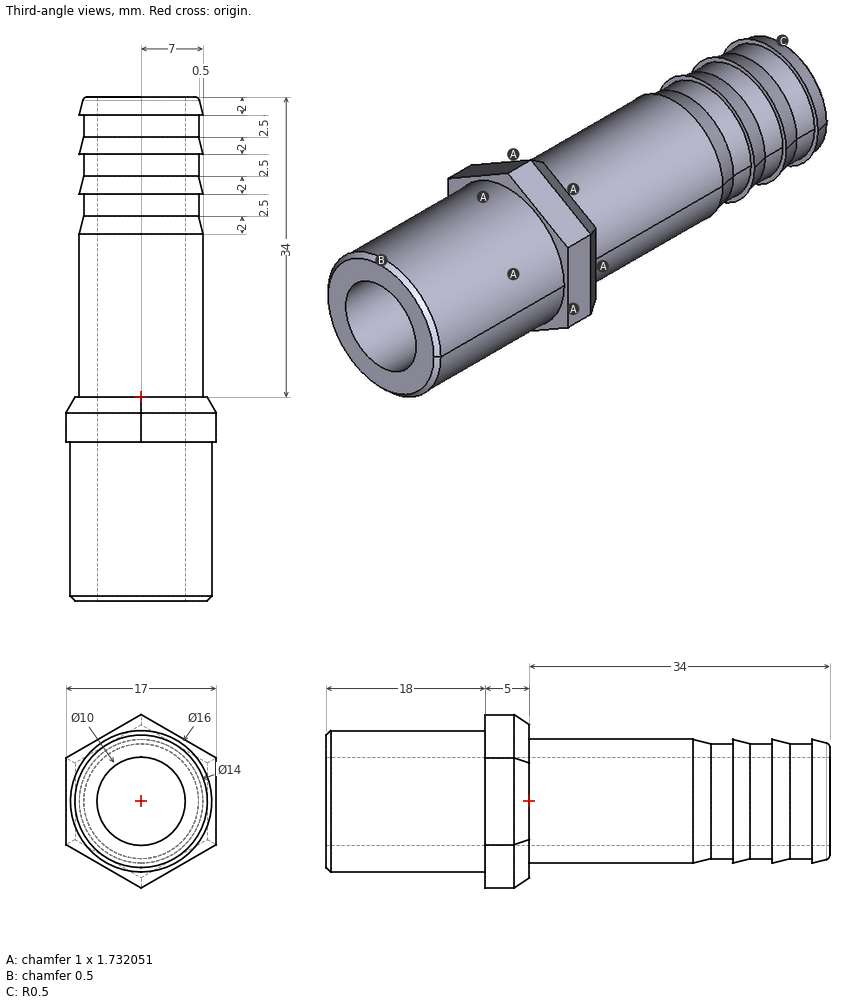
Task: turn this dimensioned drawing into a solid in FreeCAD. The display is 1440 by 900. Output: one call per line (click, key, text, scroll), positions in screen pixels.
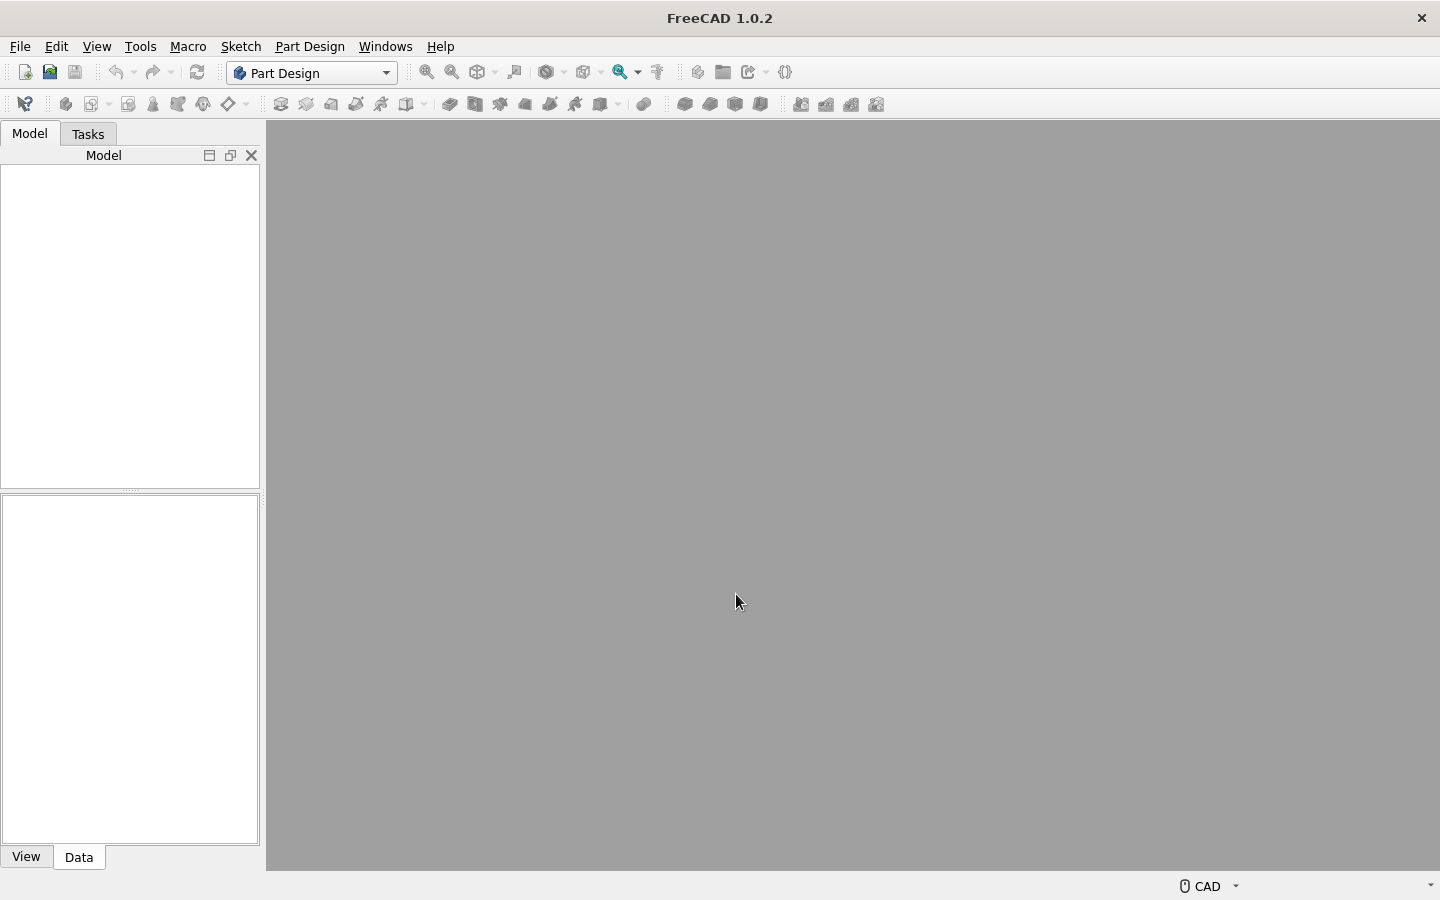
click(25, 72)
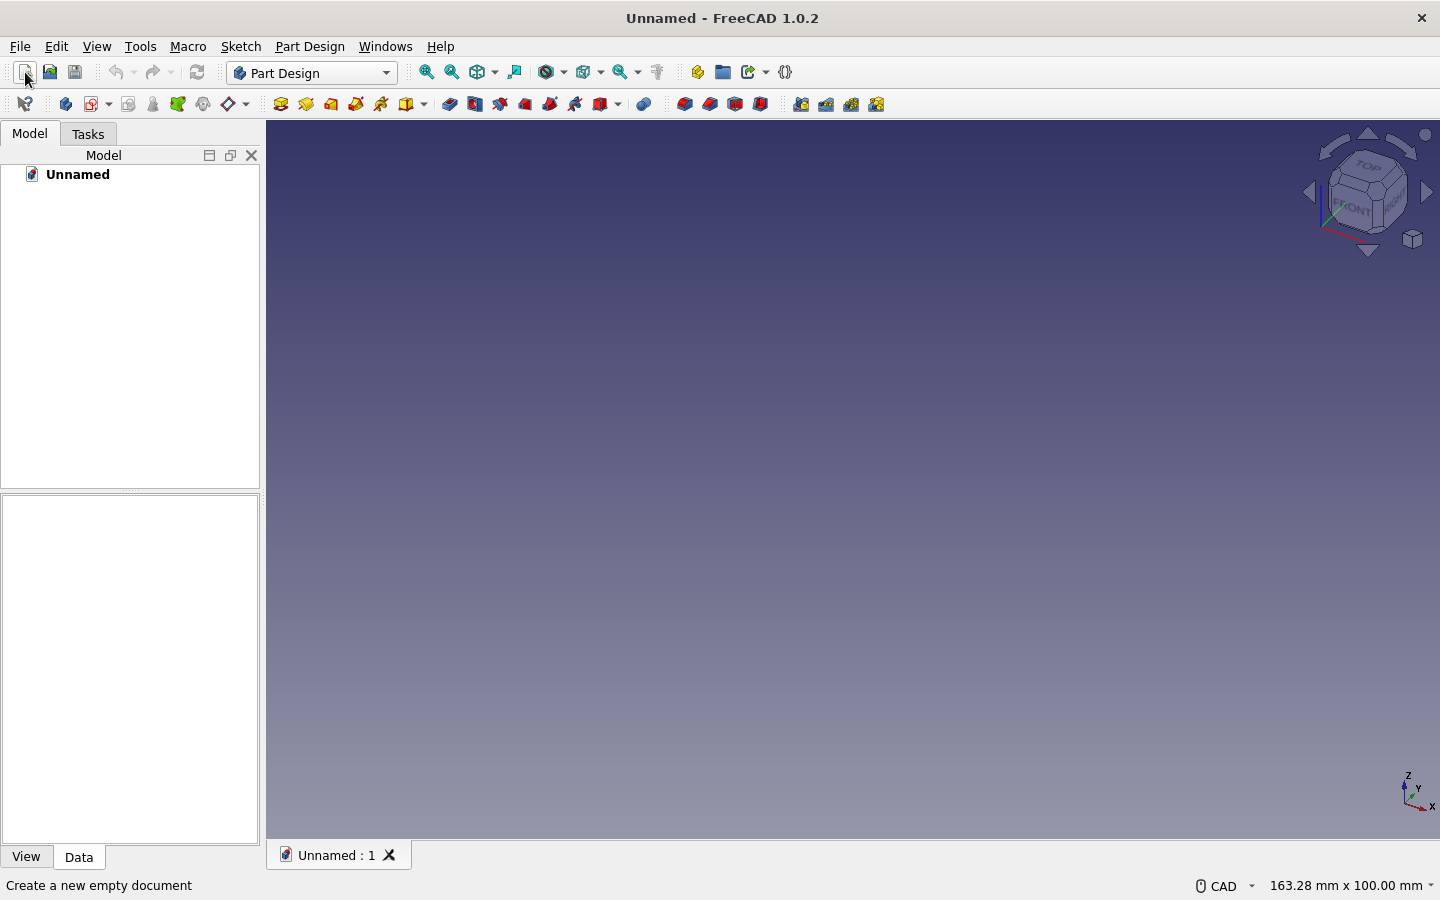
click(90, 104)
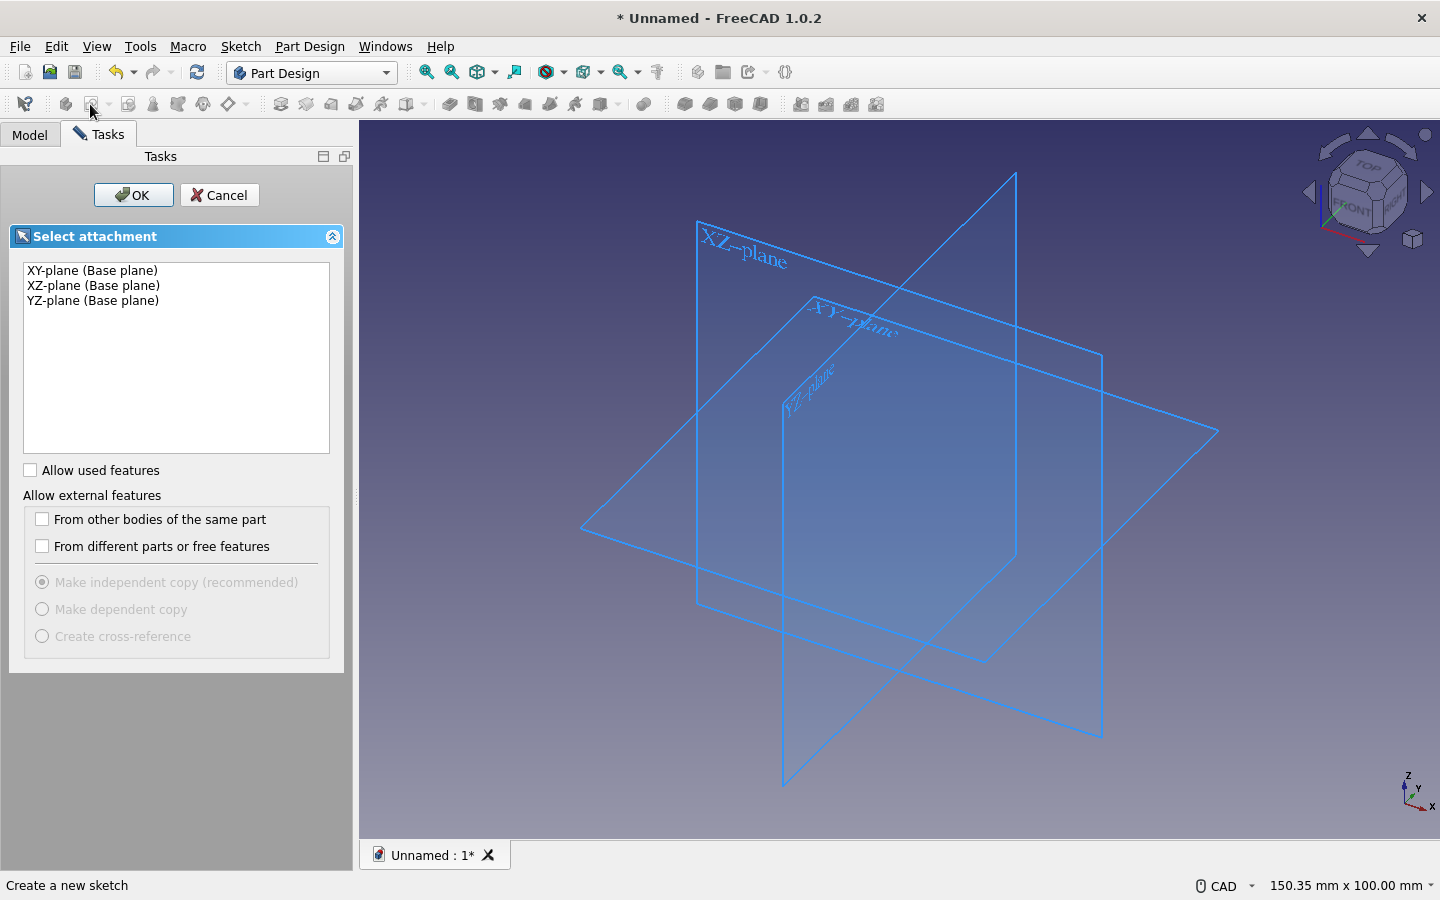
click(84, 286)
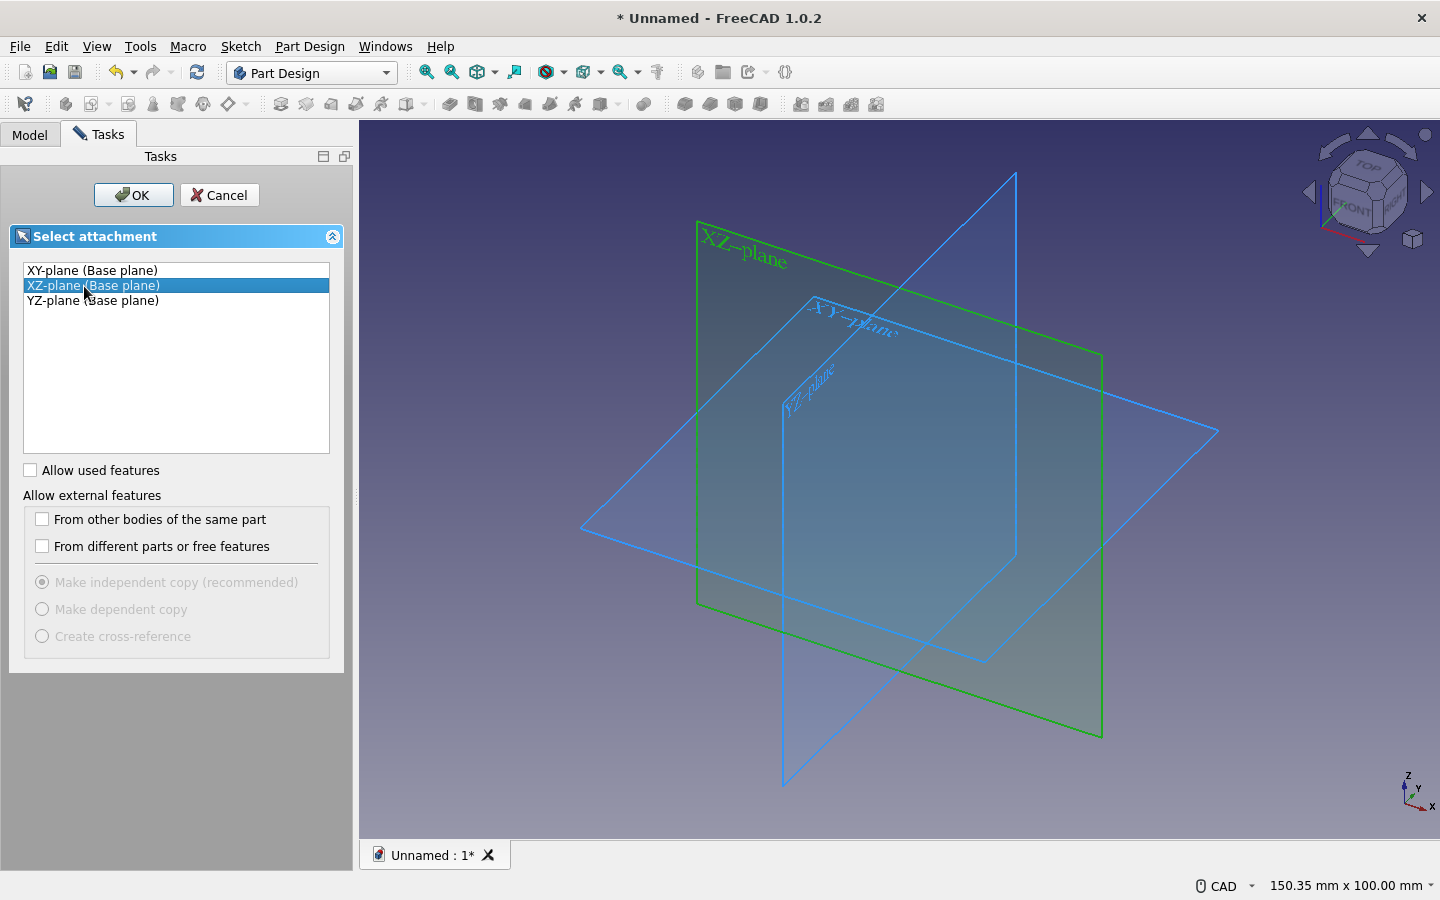
click(134, 195)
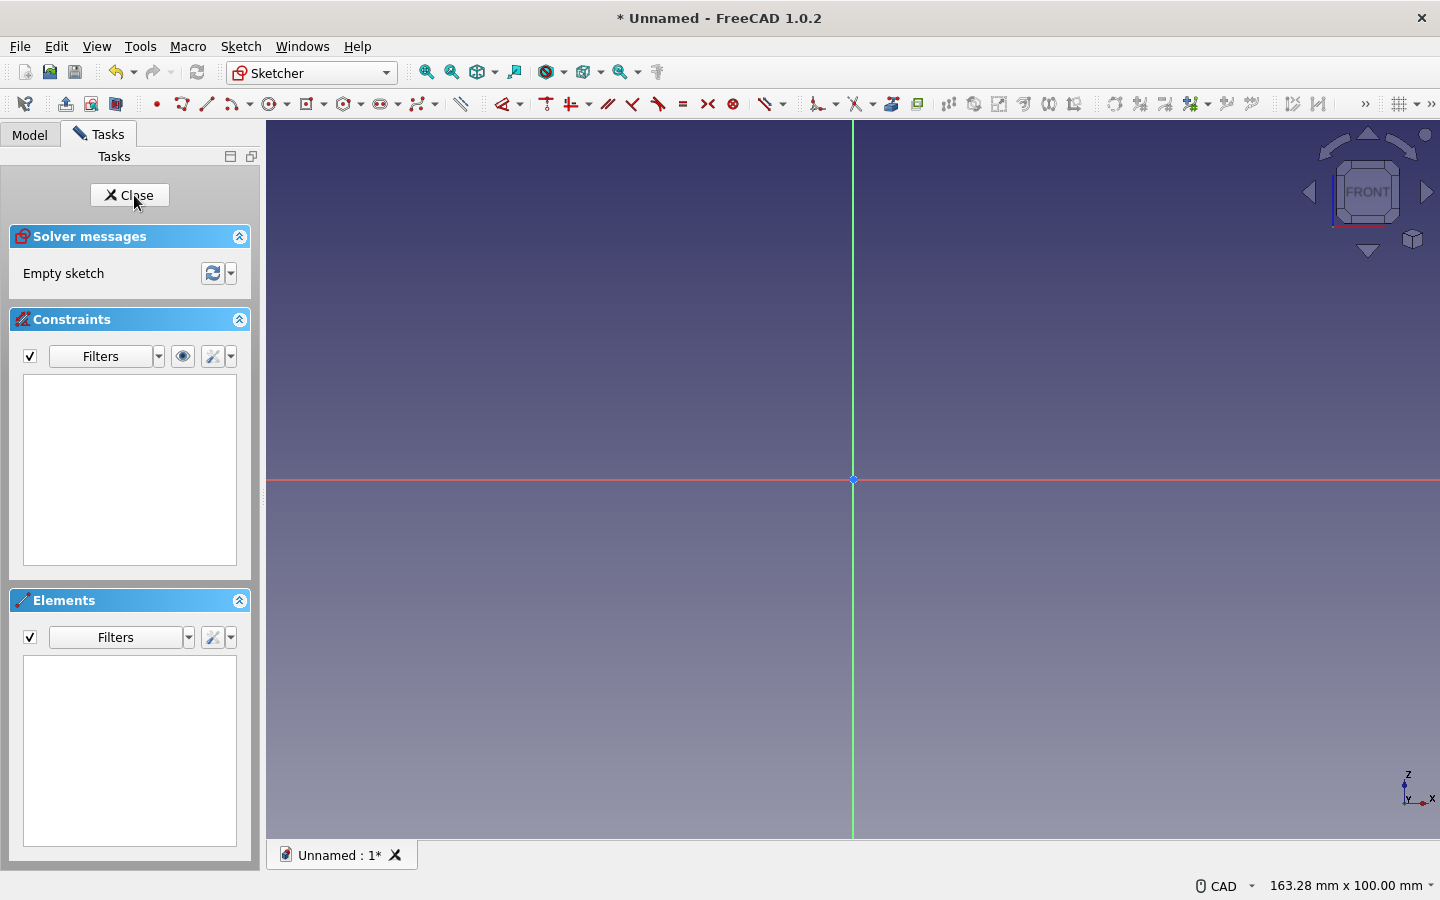
scroll(870, 479, up, 8)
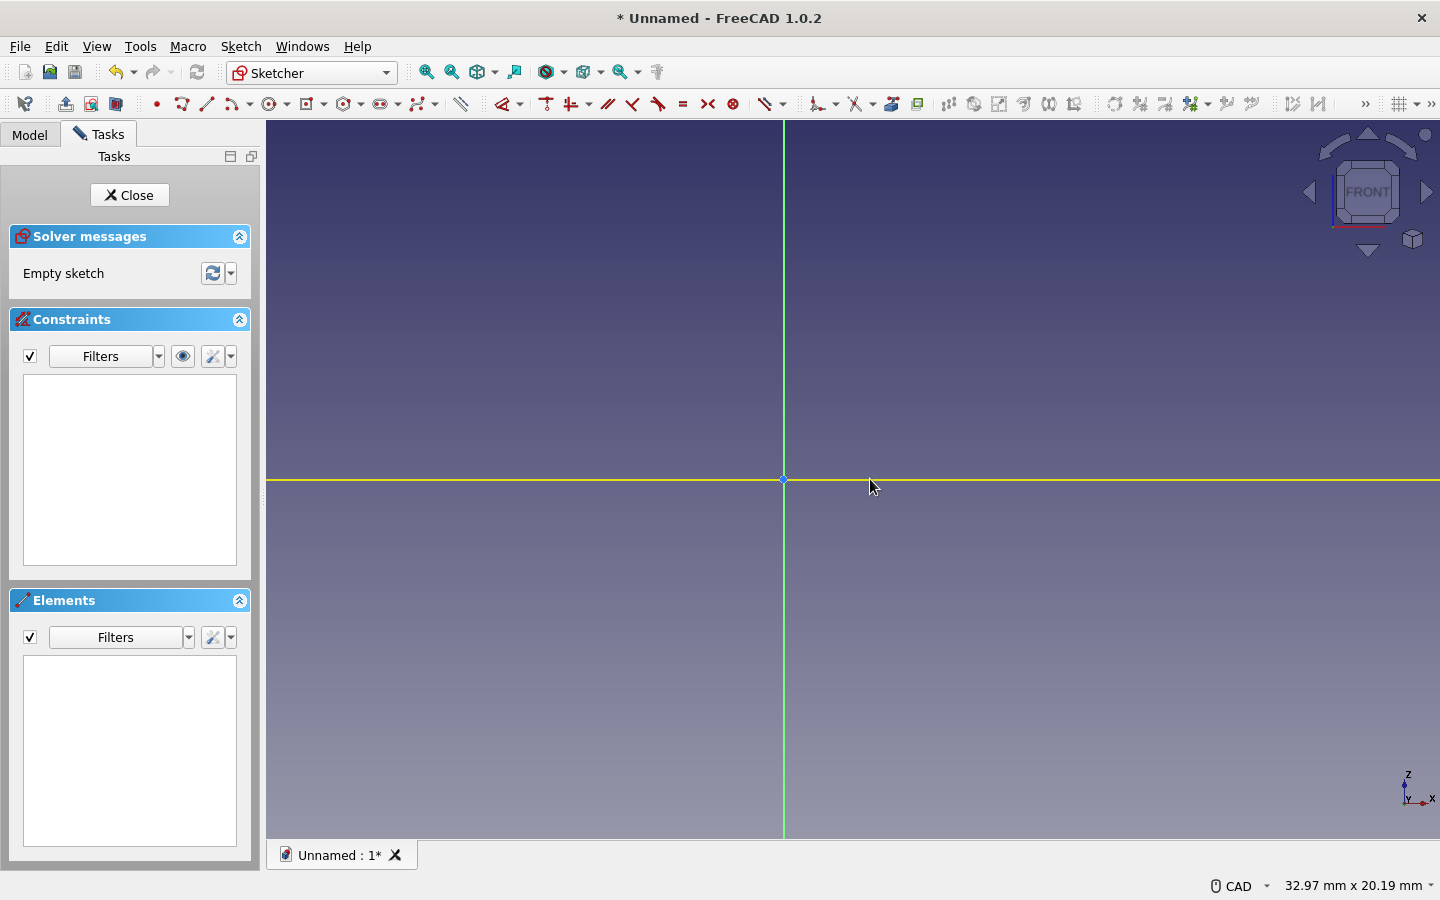
click(268, 104)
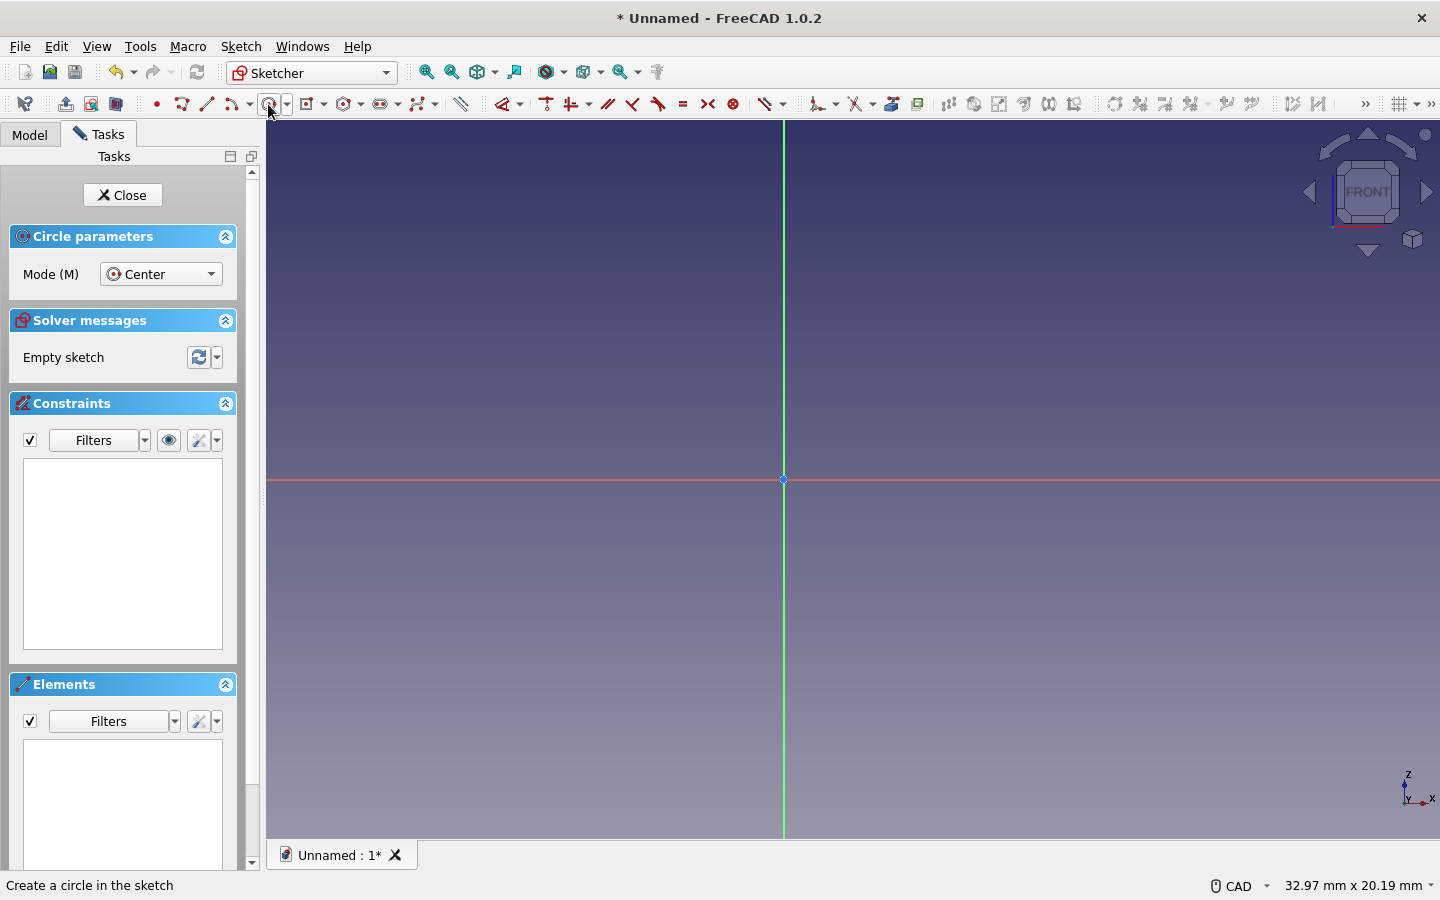
click(784, 480)
click(960, 303)
key(Escape)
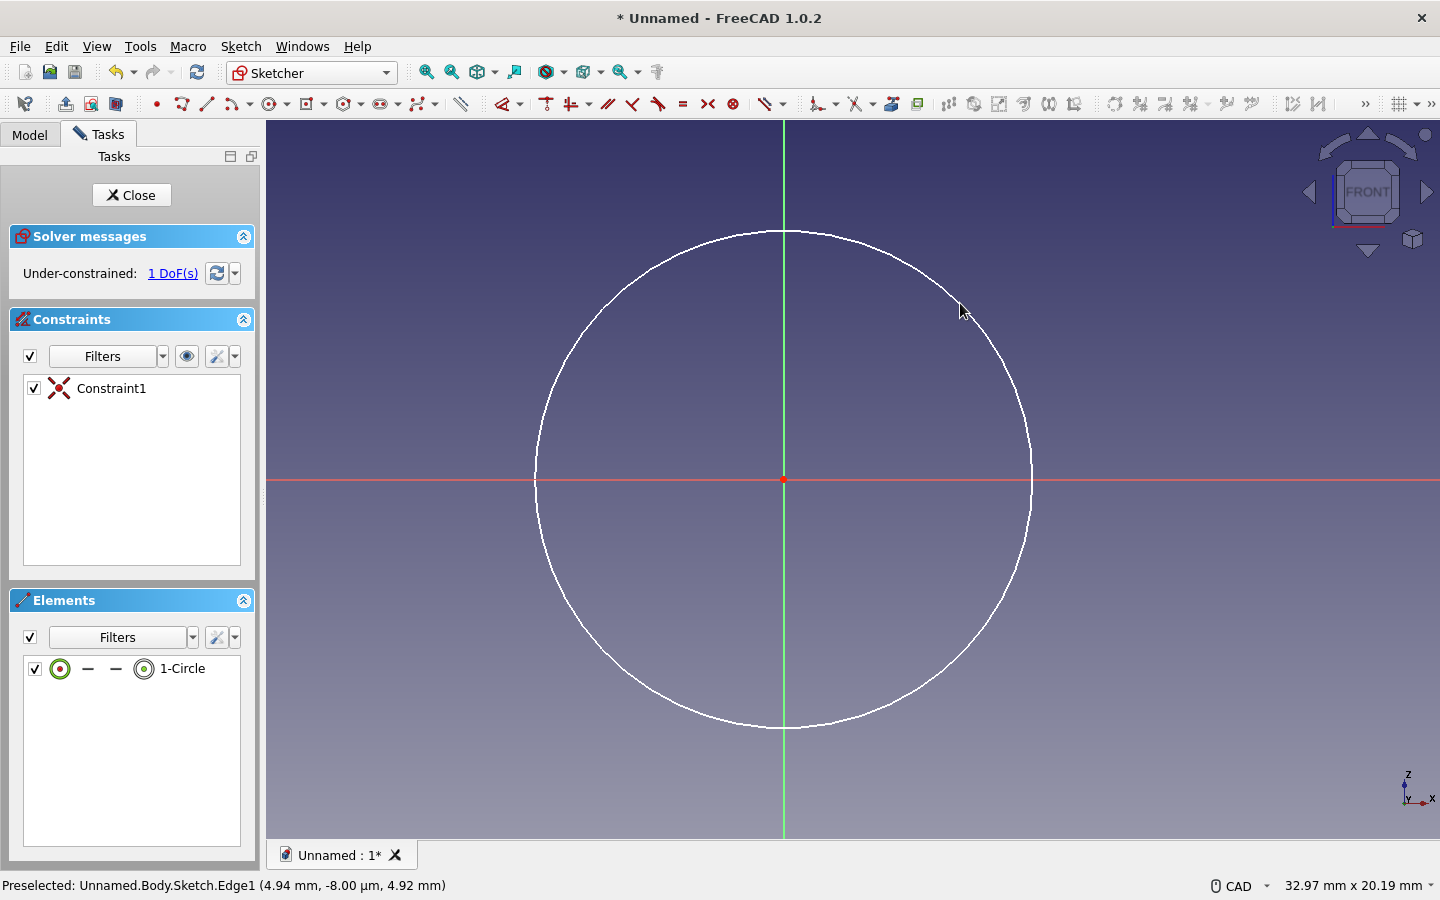
click(502, 104)